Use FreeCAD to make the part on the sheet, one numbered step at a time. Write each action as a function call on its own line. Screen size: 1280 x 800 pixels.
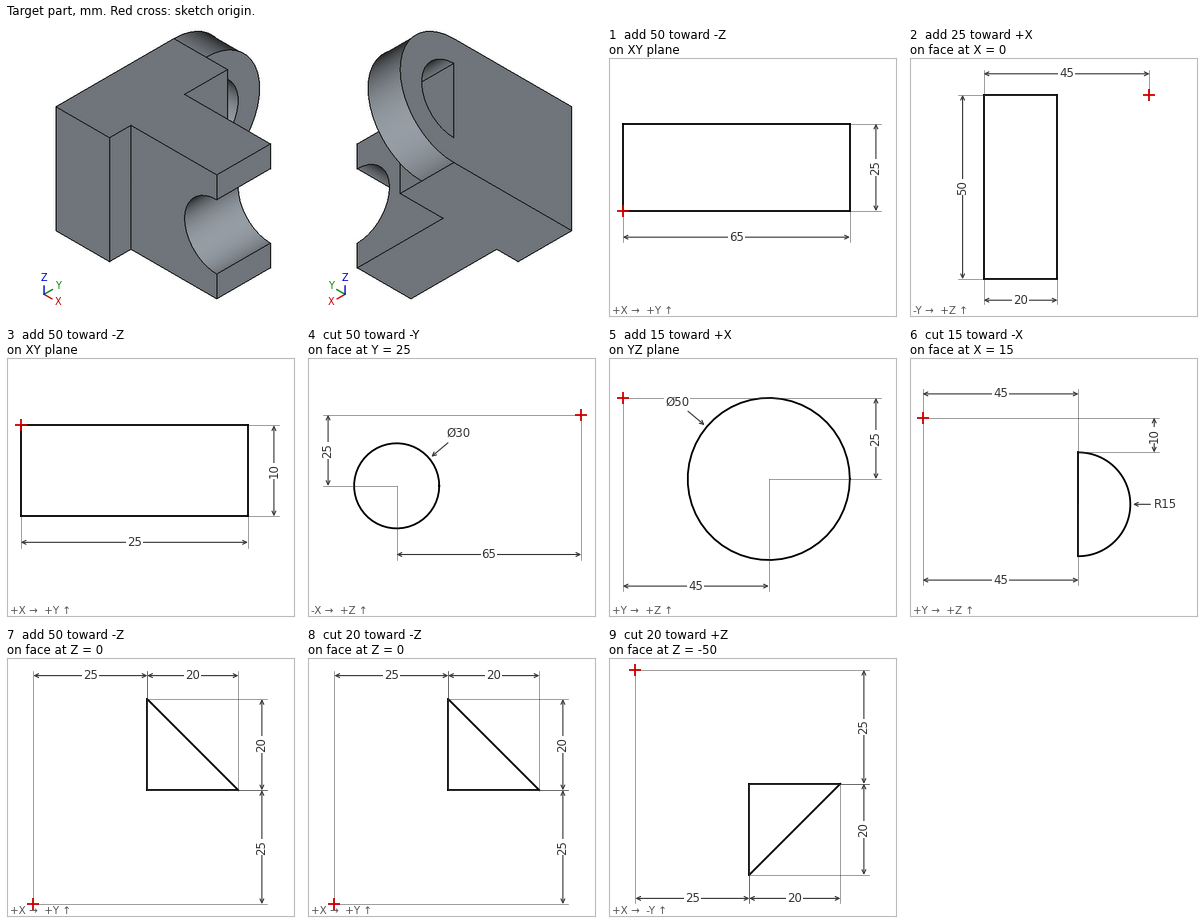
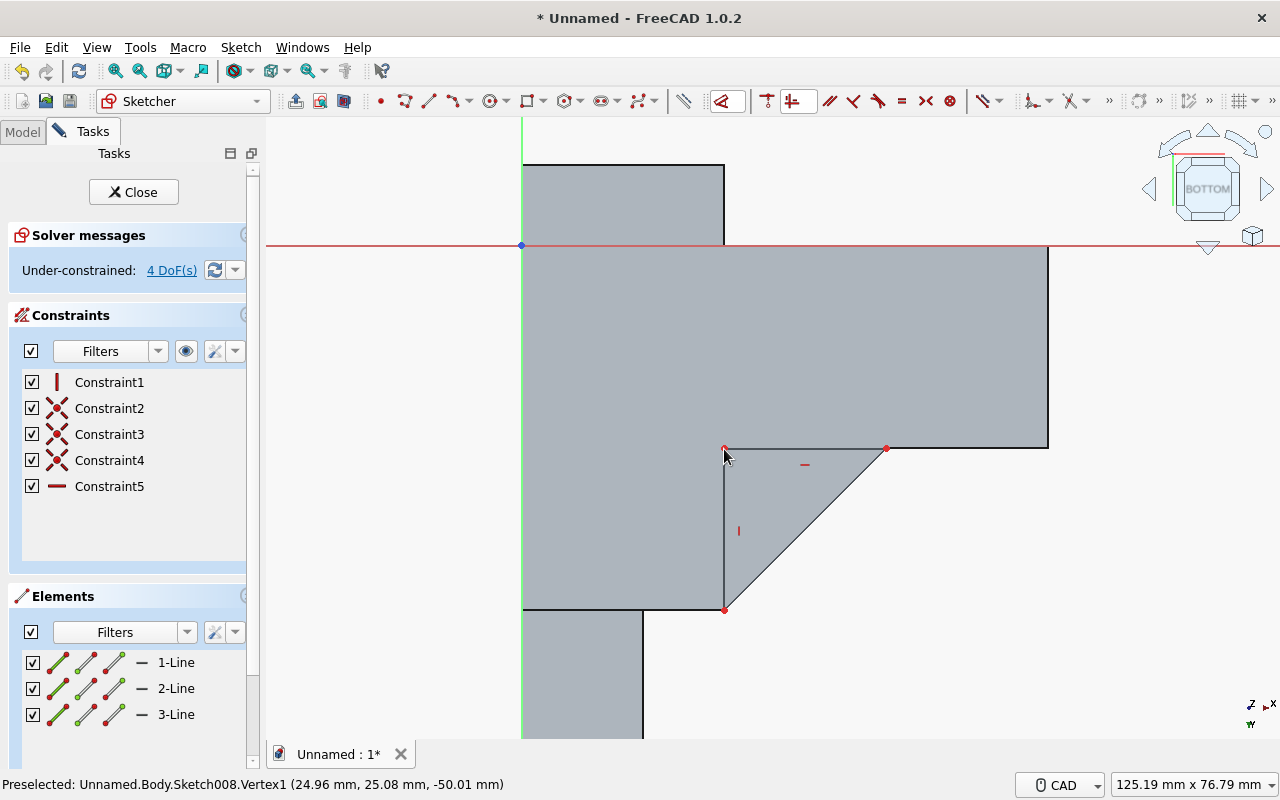
click(724, 498)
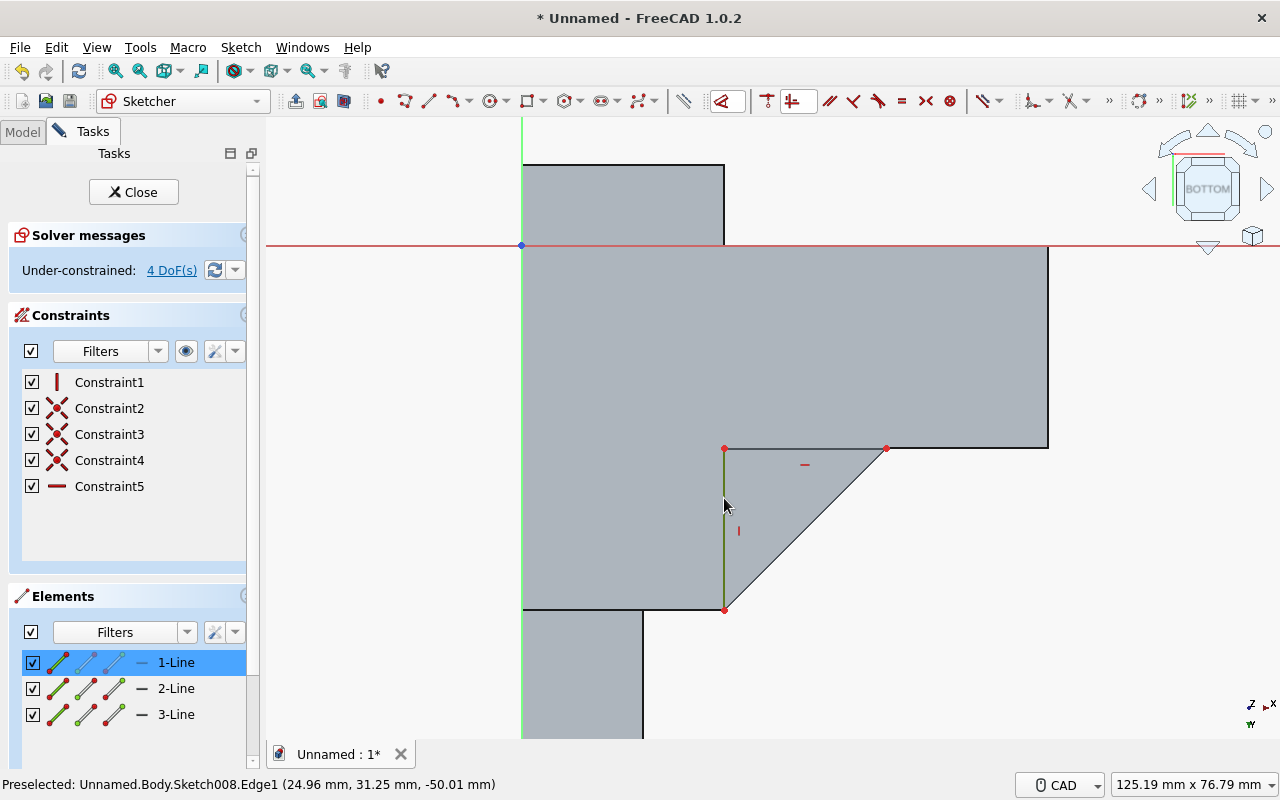
key(i)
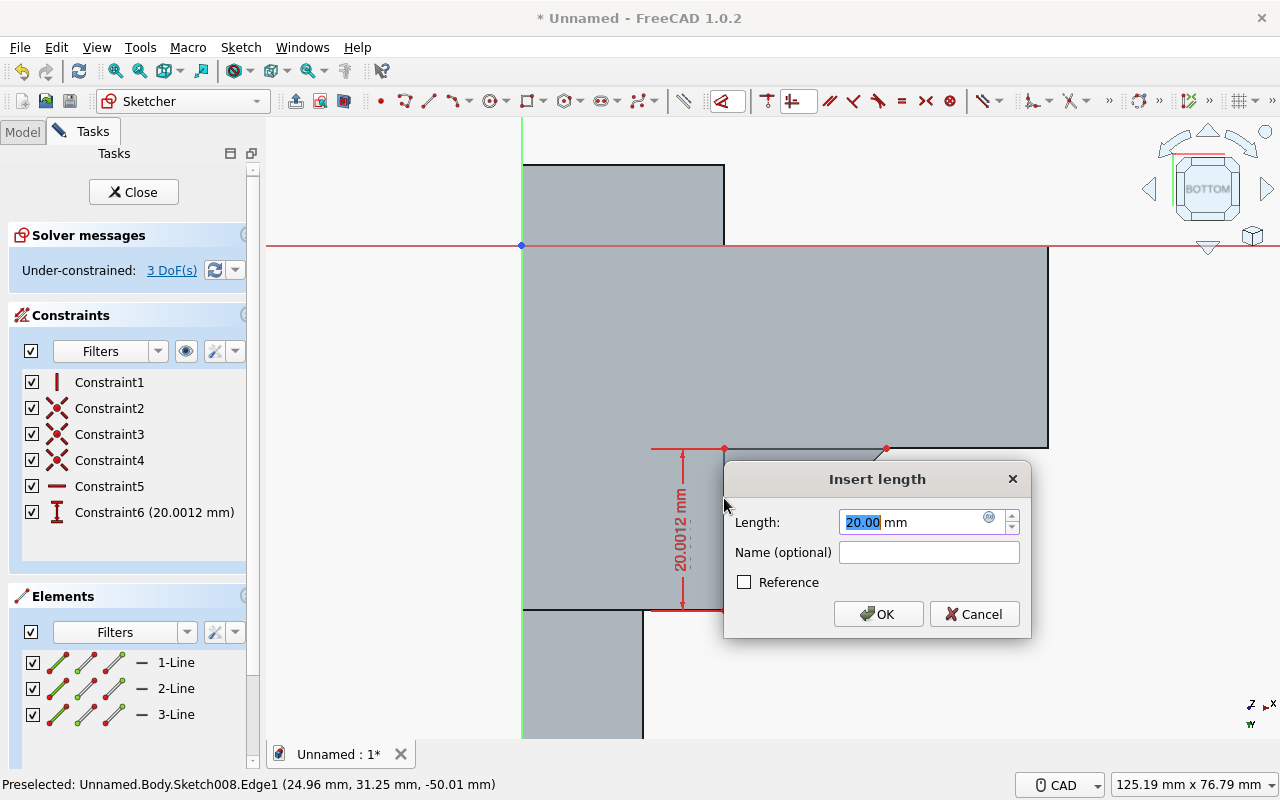
text(20)
key(Return)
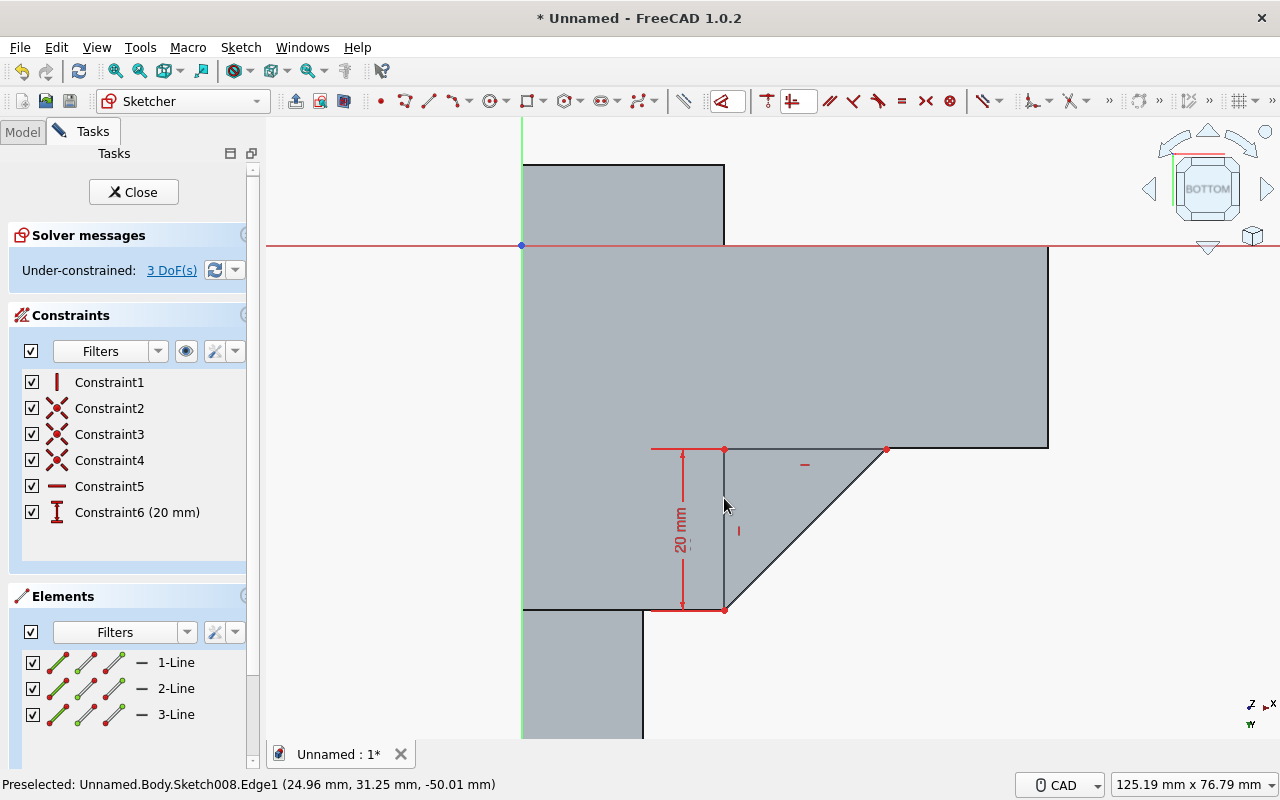
click(837, 449)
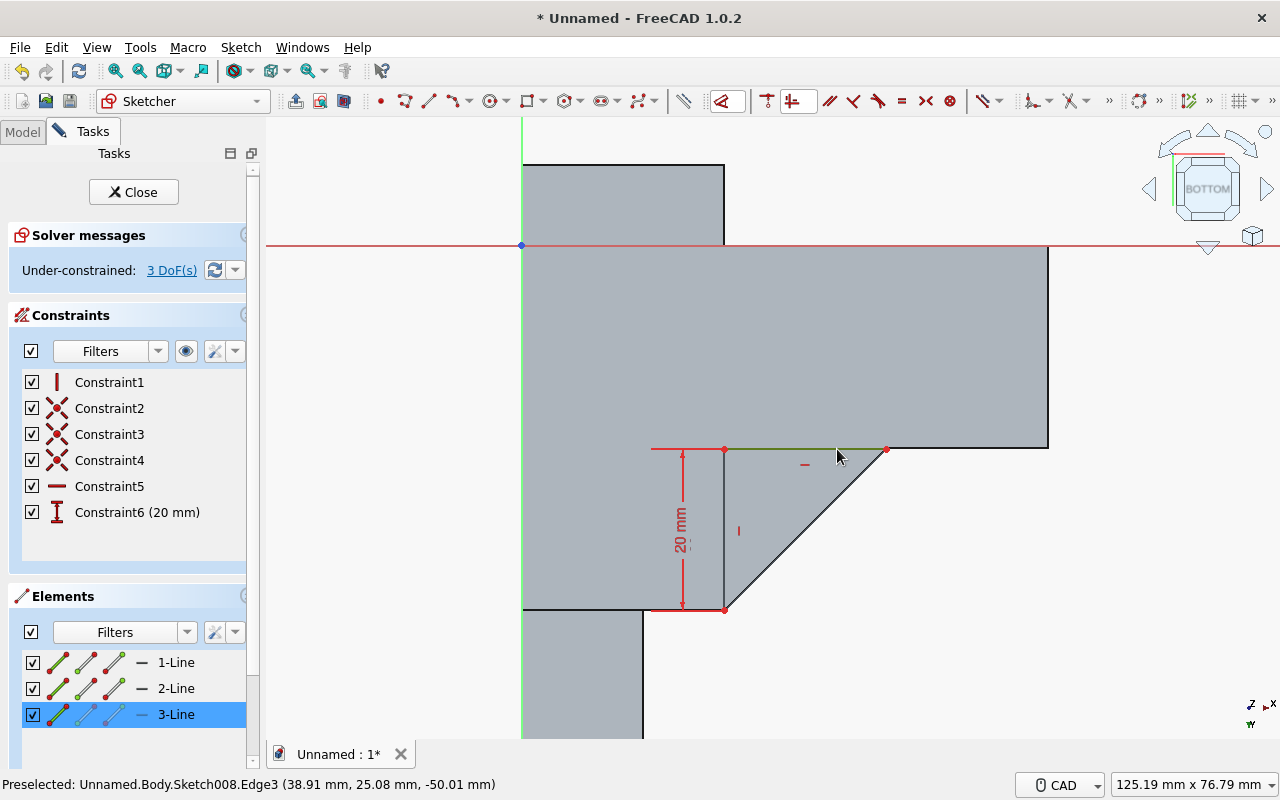
key(l)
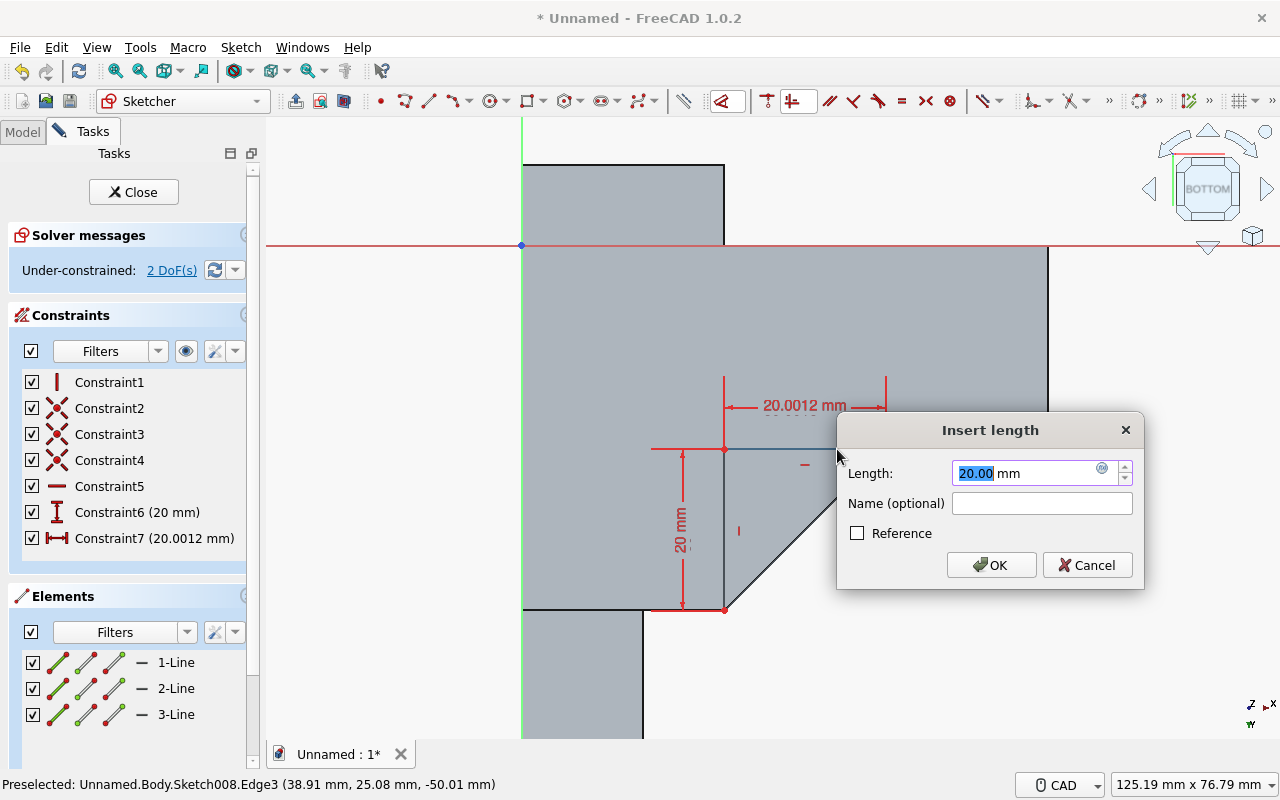
text(20)
key(Return)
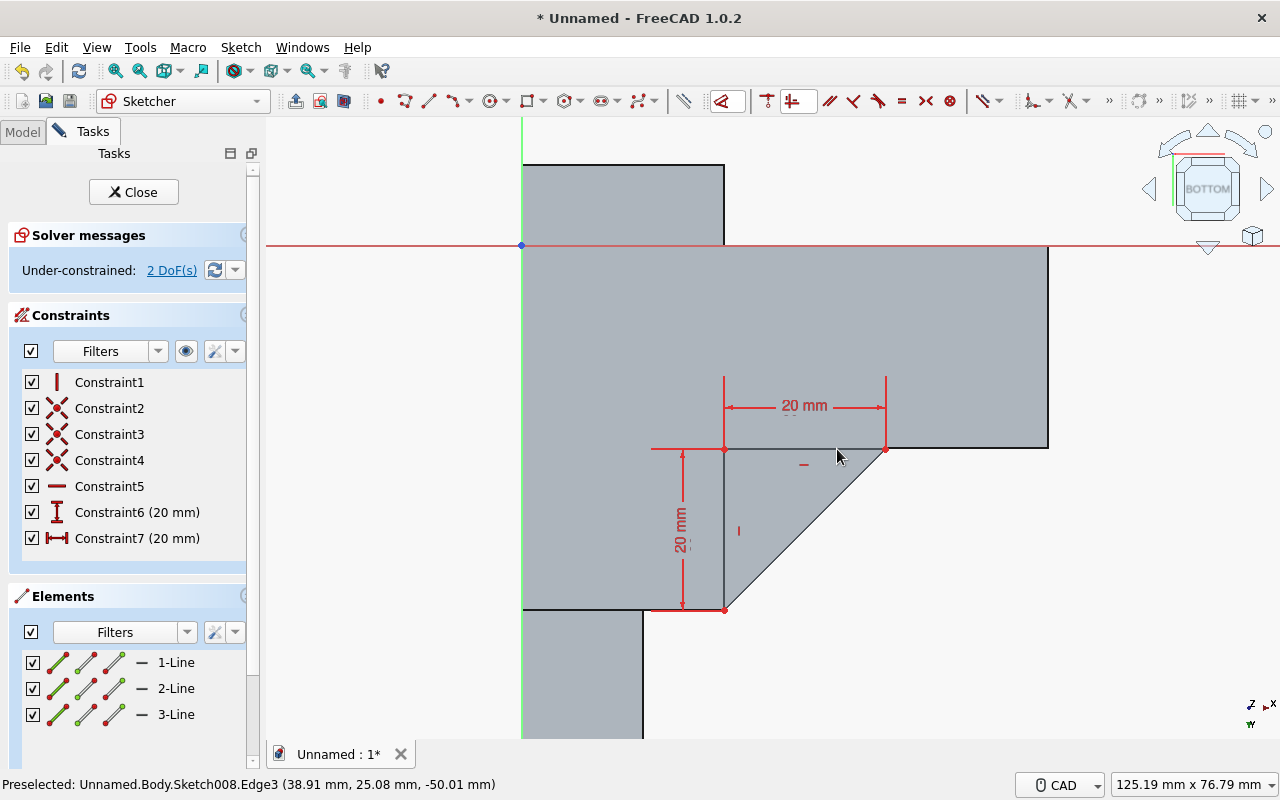
click(724, 449)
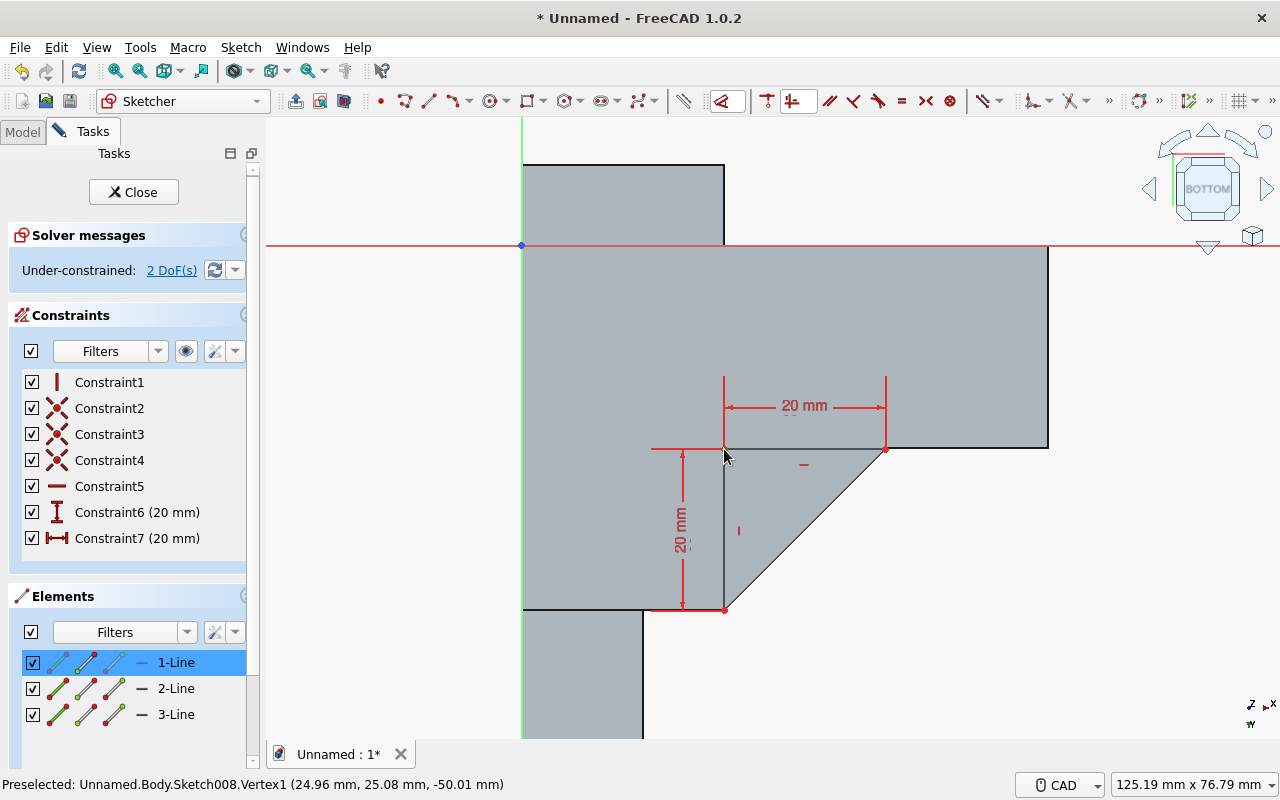
key(l)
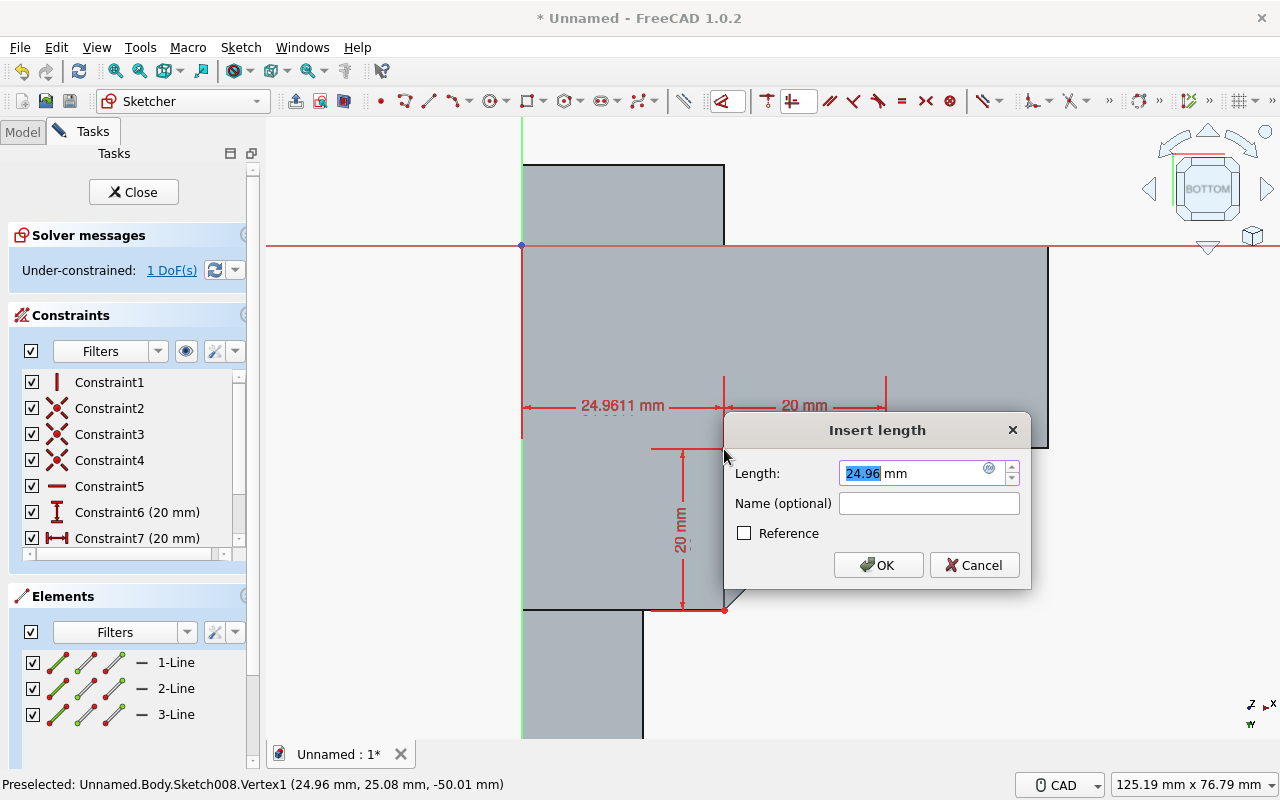
text(25)
key(Return)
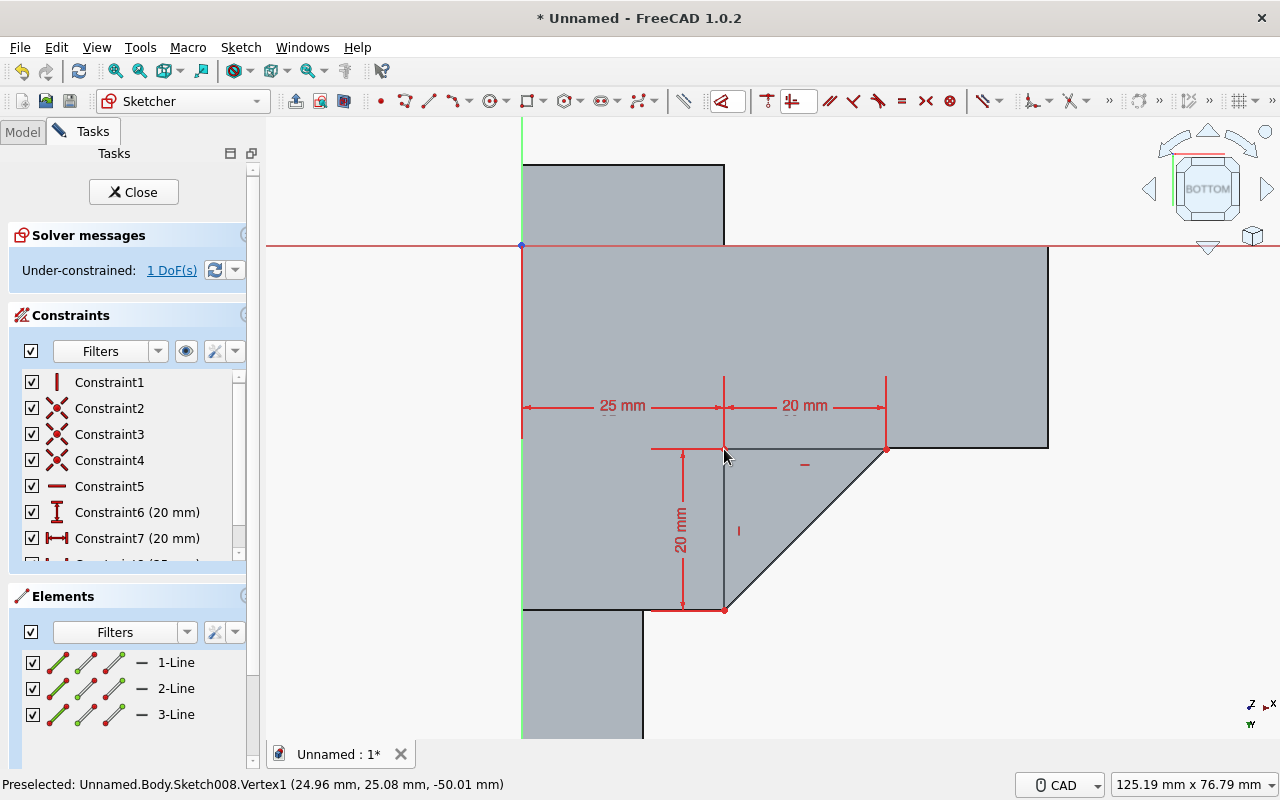
click(724, 449)